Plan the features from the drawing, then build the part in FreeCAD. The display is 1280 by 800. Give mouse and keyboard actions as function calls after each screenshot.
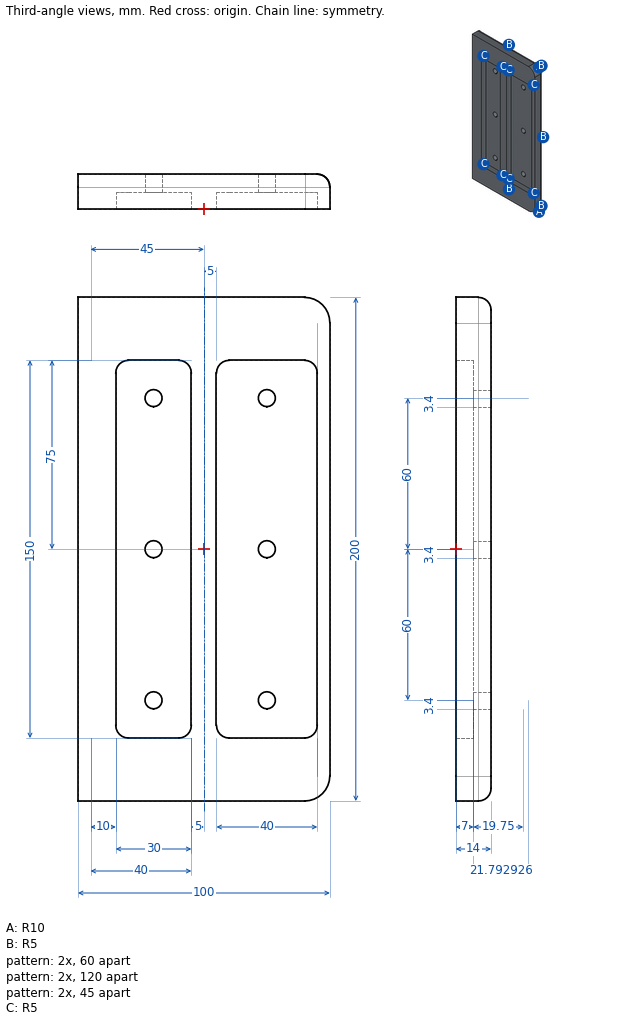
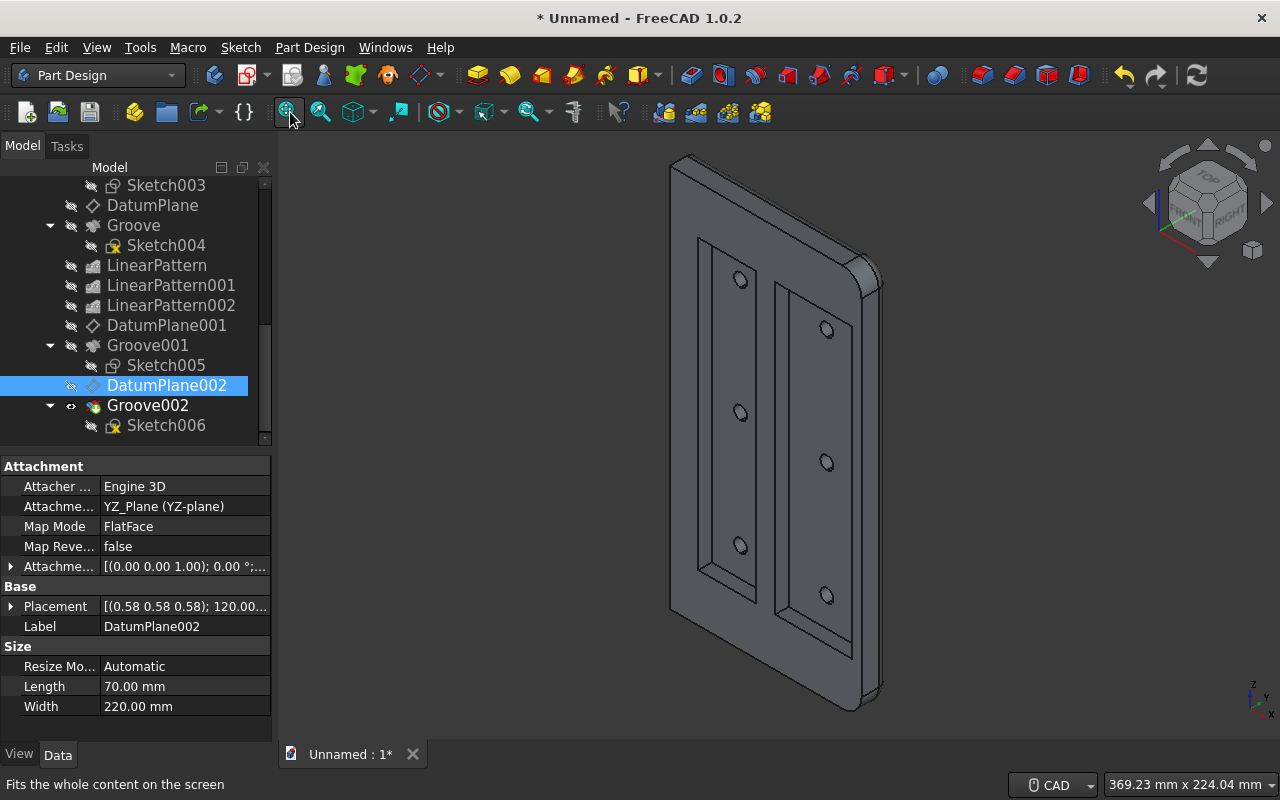
key(1)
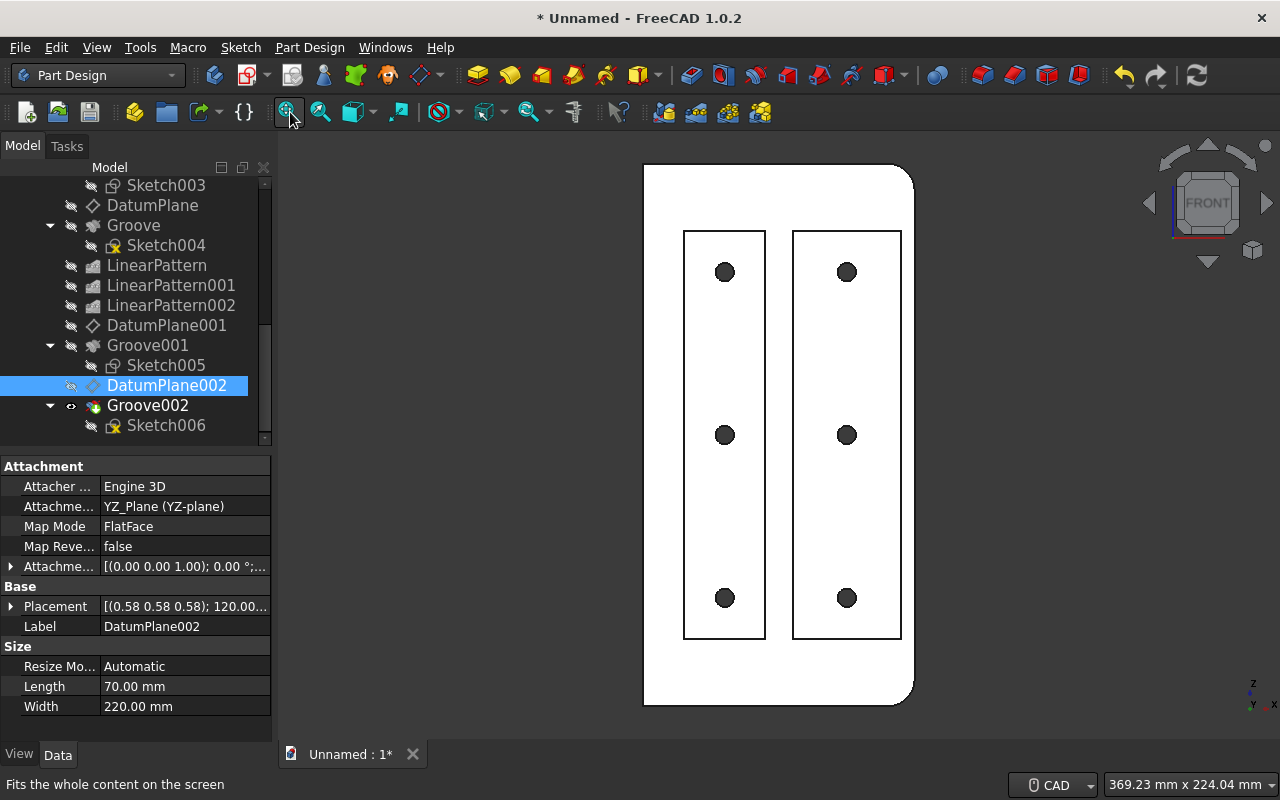
scroll(901, 230, up, 4)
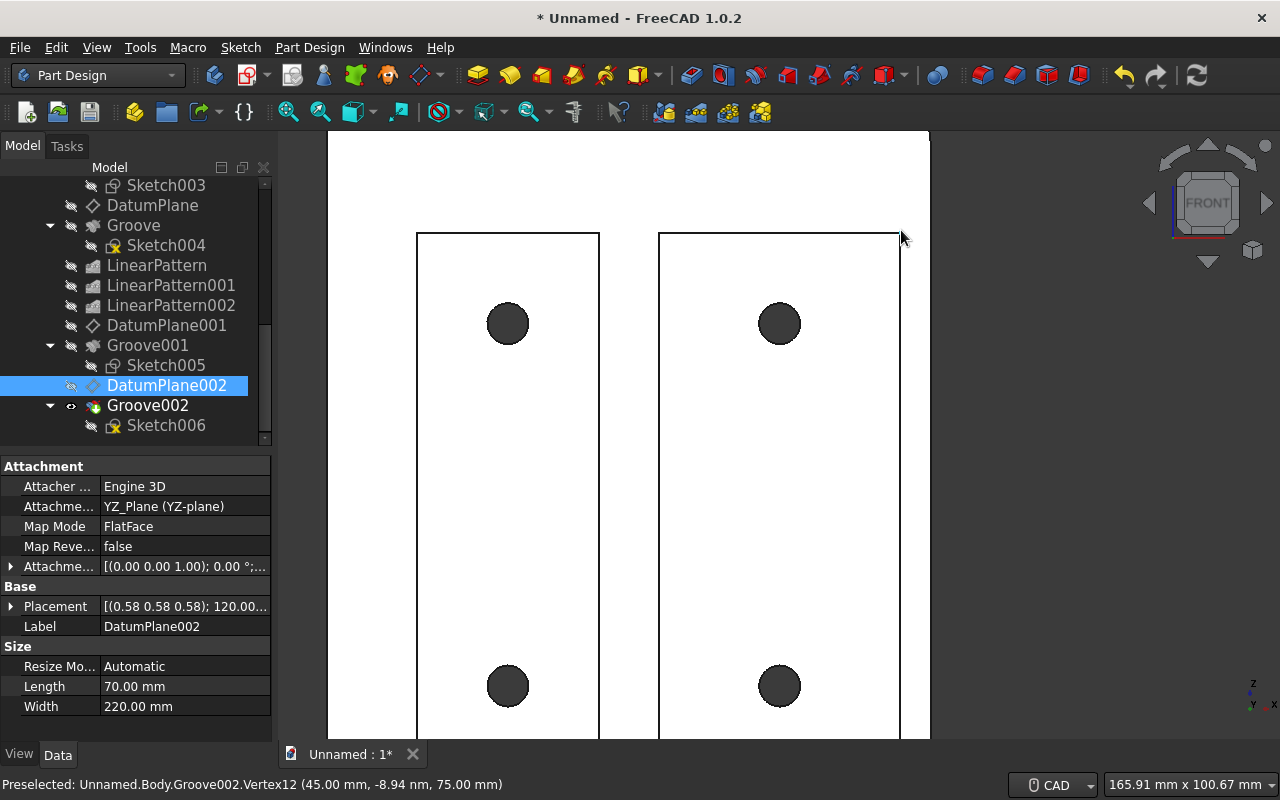
click(290, 112)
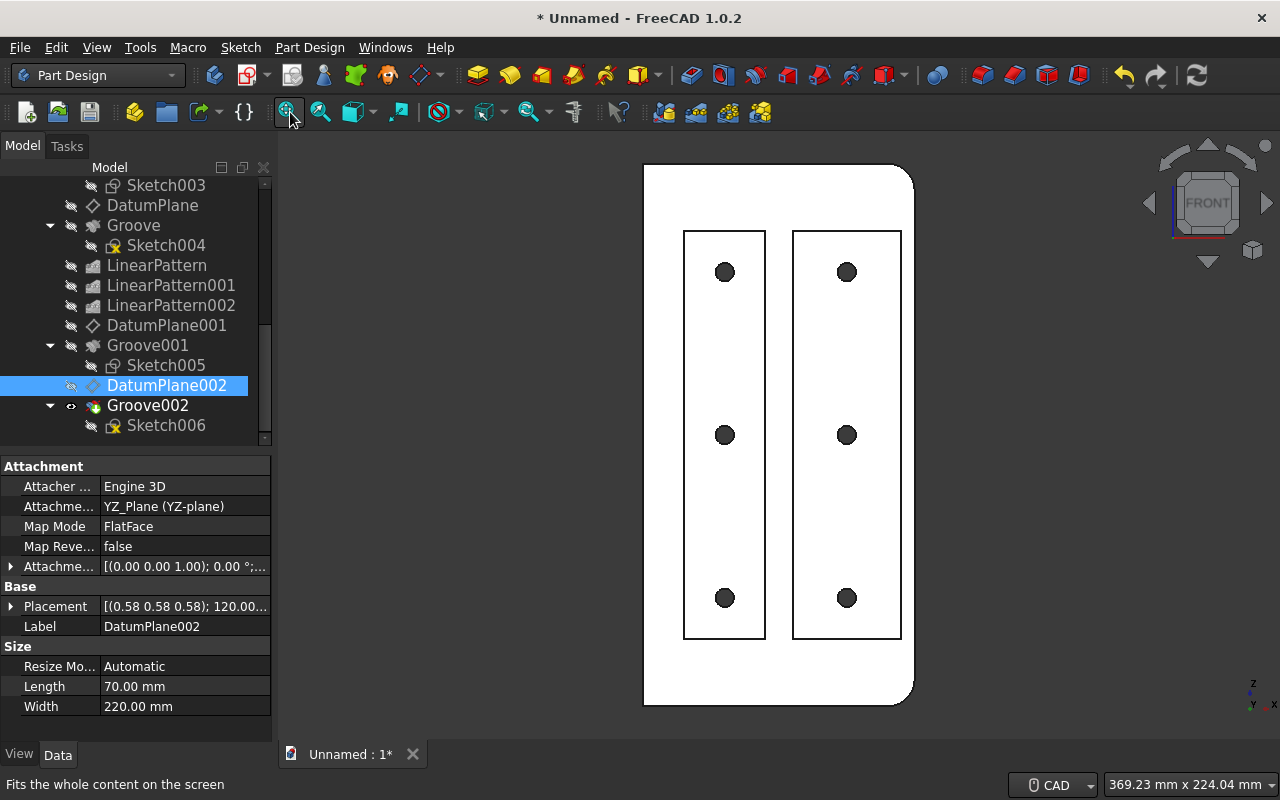
key(3)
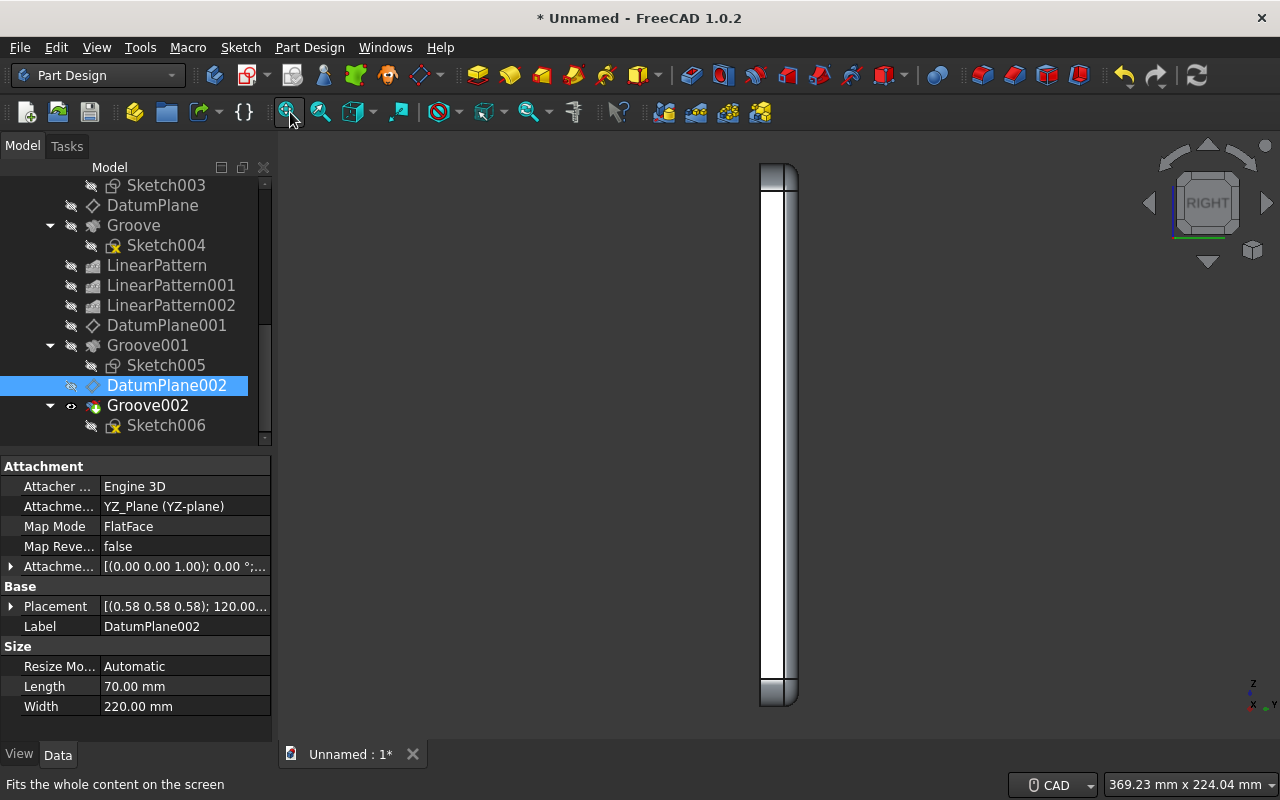
scroll(770, 230, up, 4)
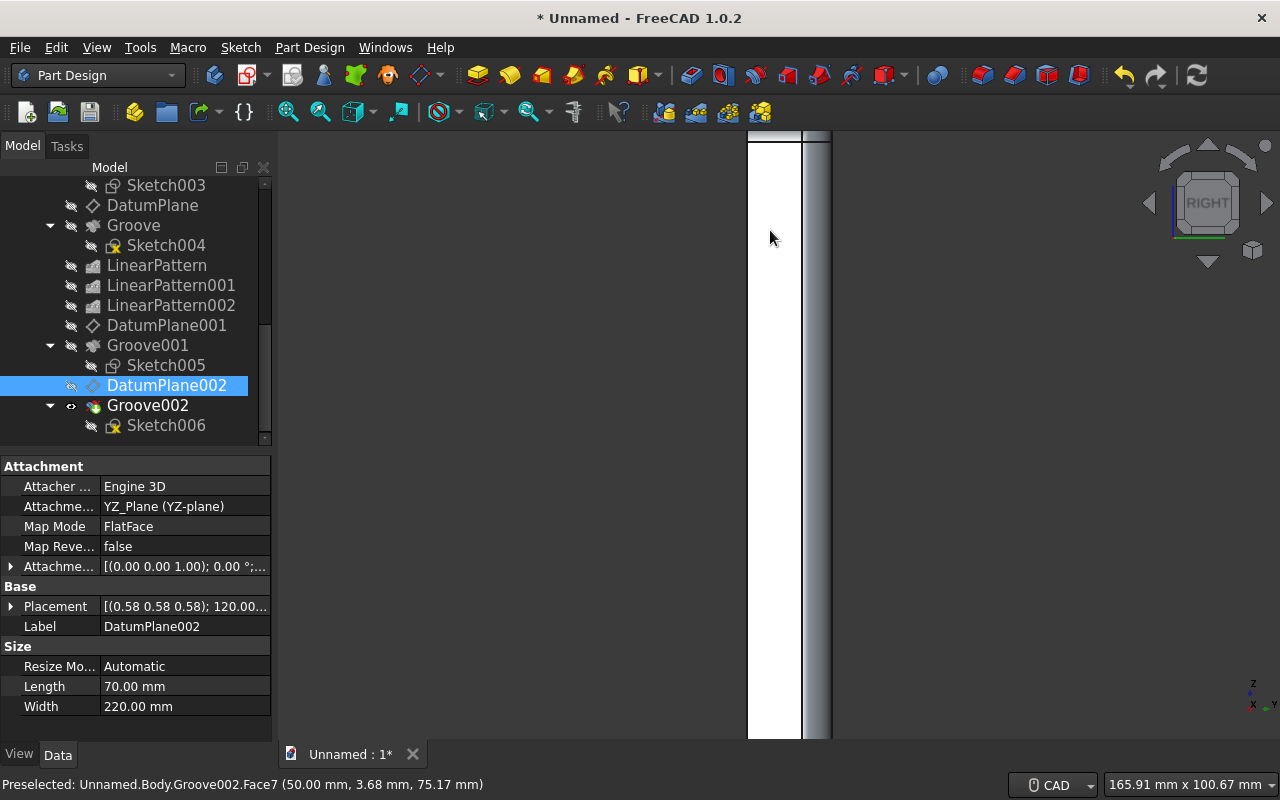
click(290, 112)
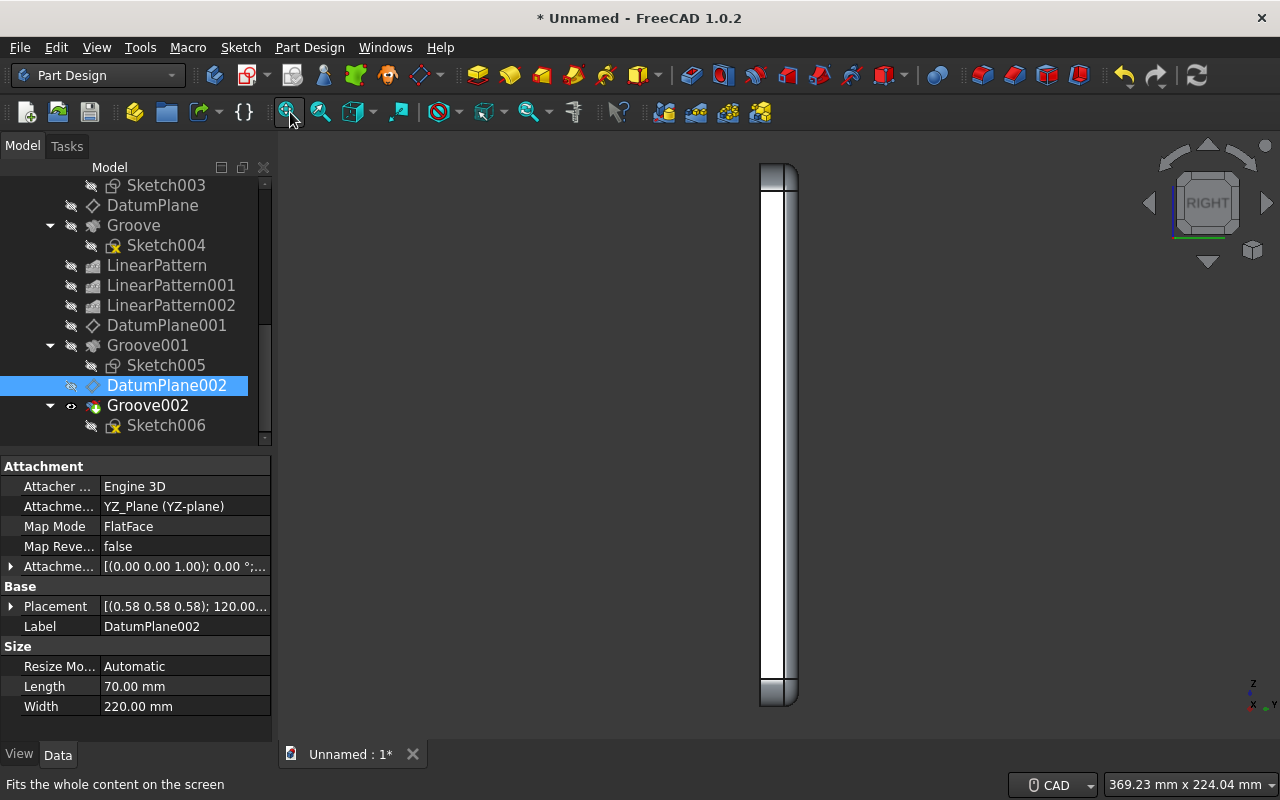
key(5)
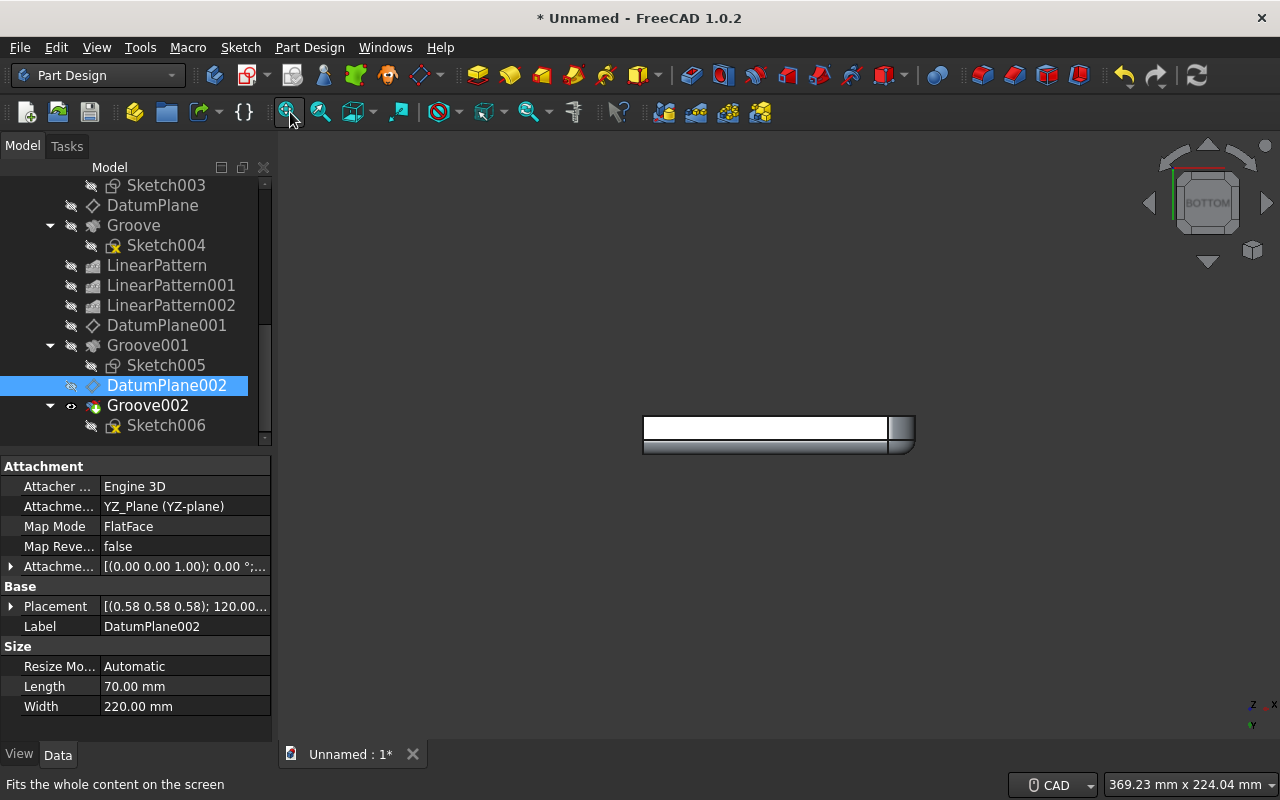
click(290, 112)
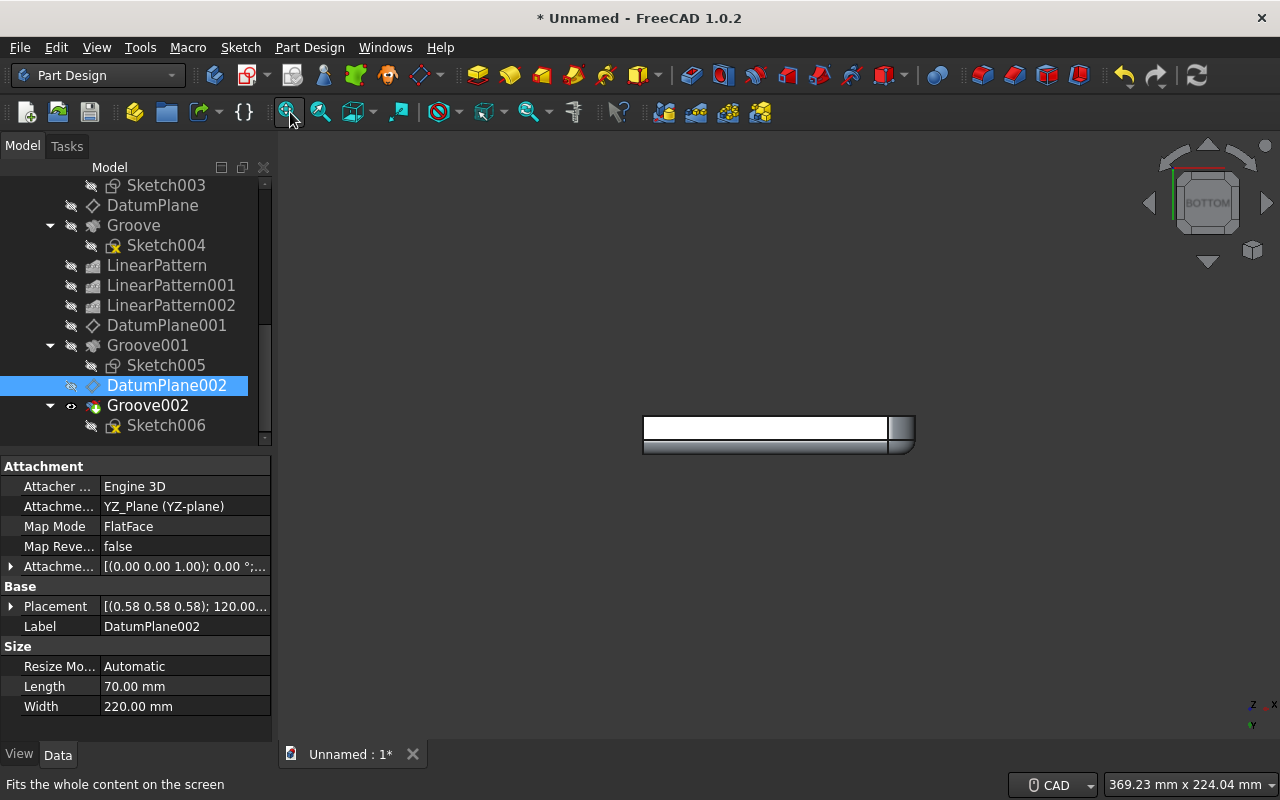
scroll(901, 425, up, 4)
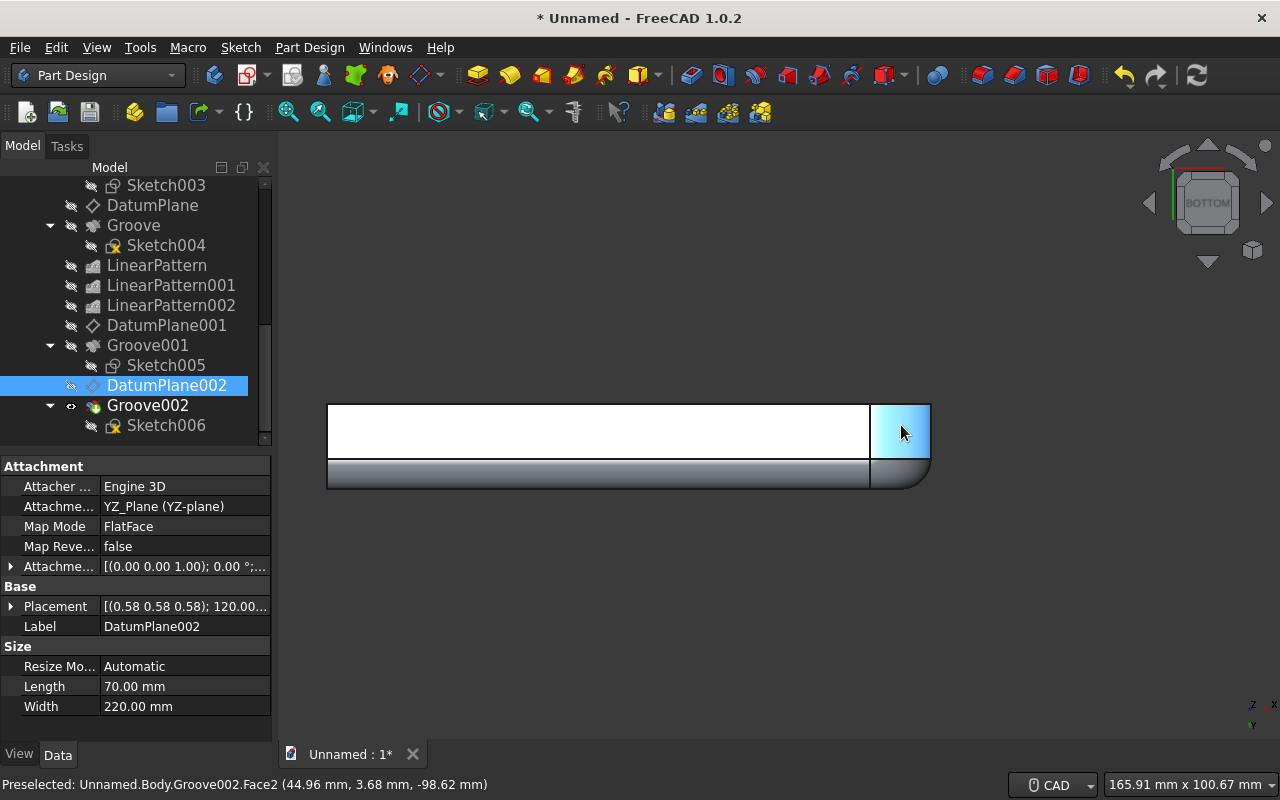
click(290, 112)